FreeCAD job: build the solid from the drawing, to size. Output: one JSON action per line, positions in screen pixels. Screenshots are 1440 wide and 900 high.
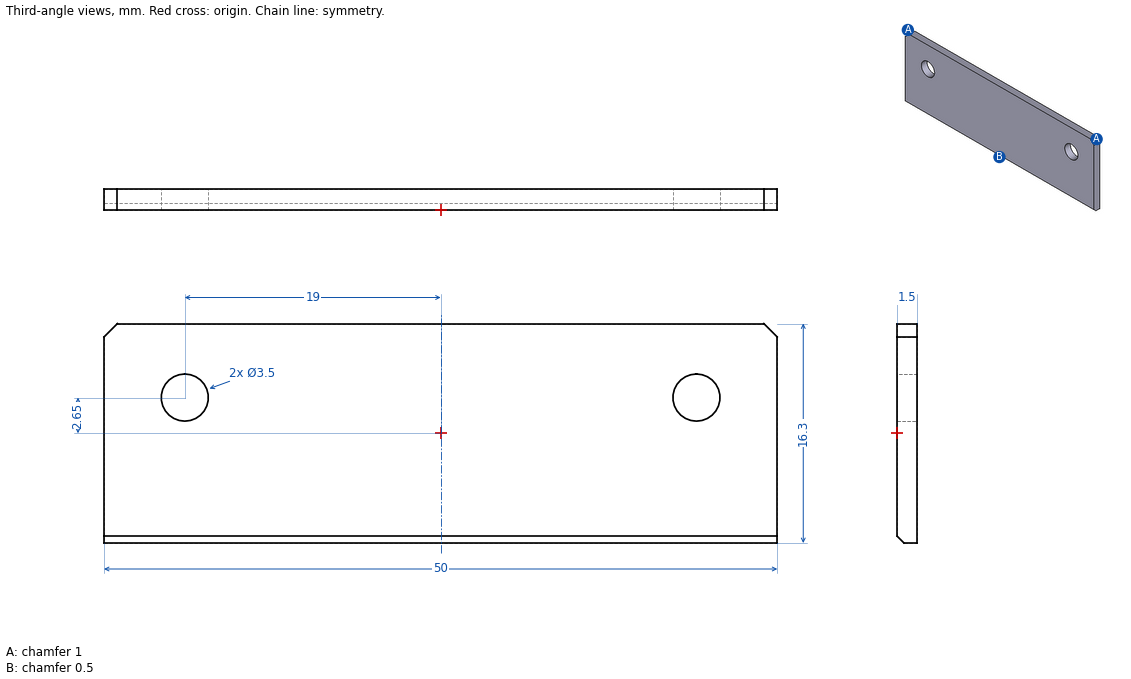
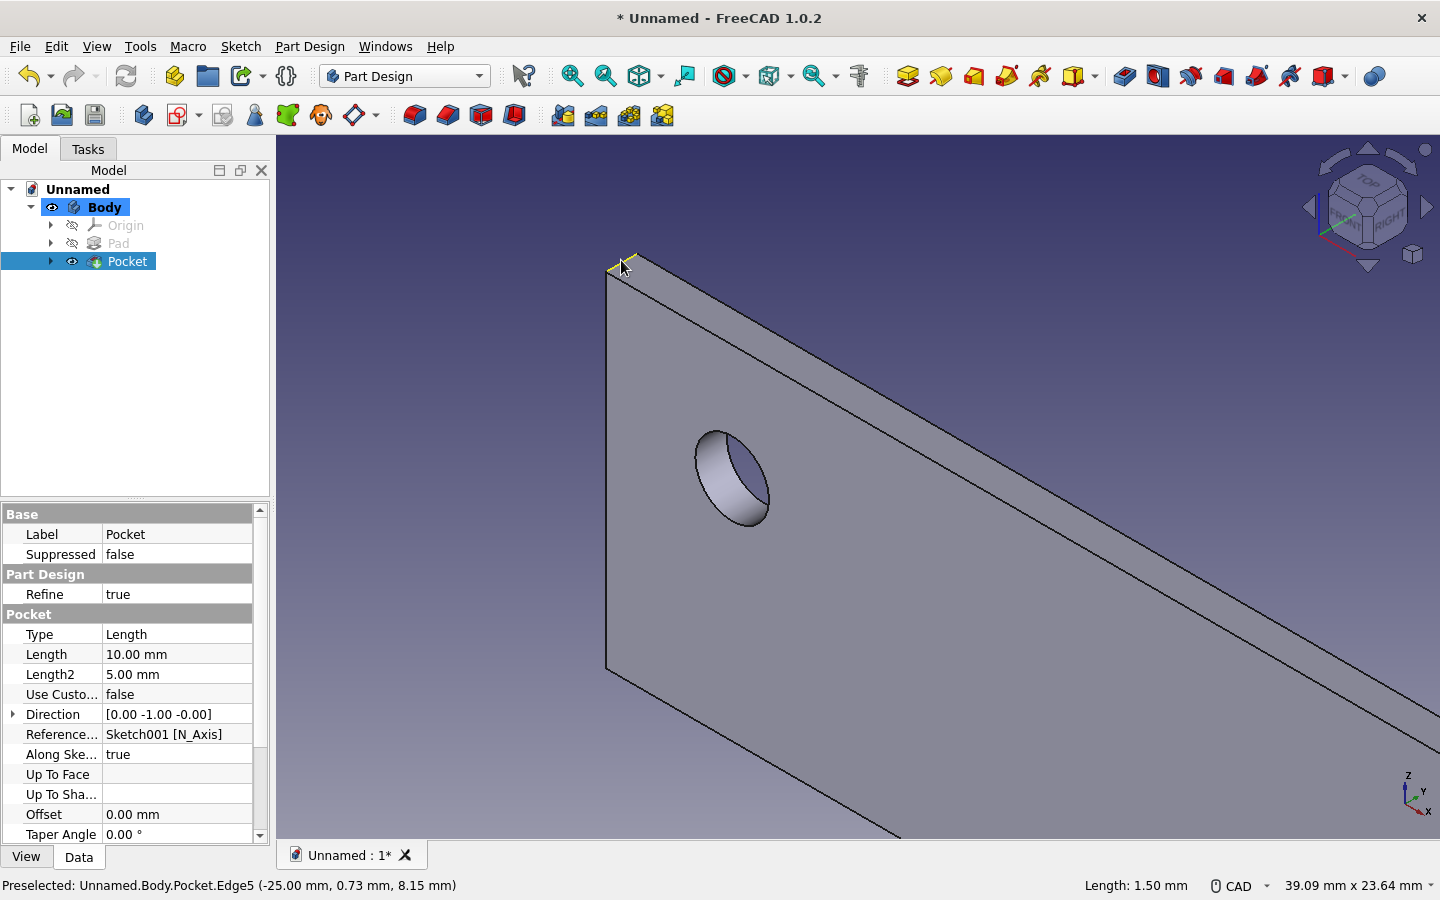
{"action": "key", "text": "v f"}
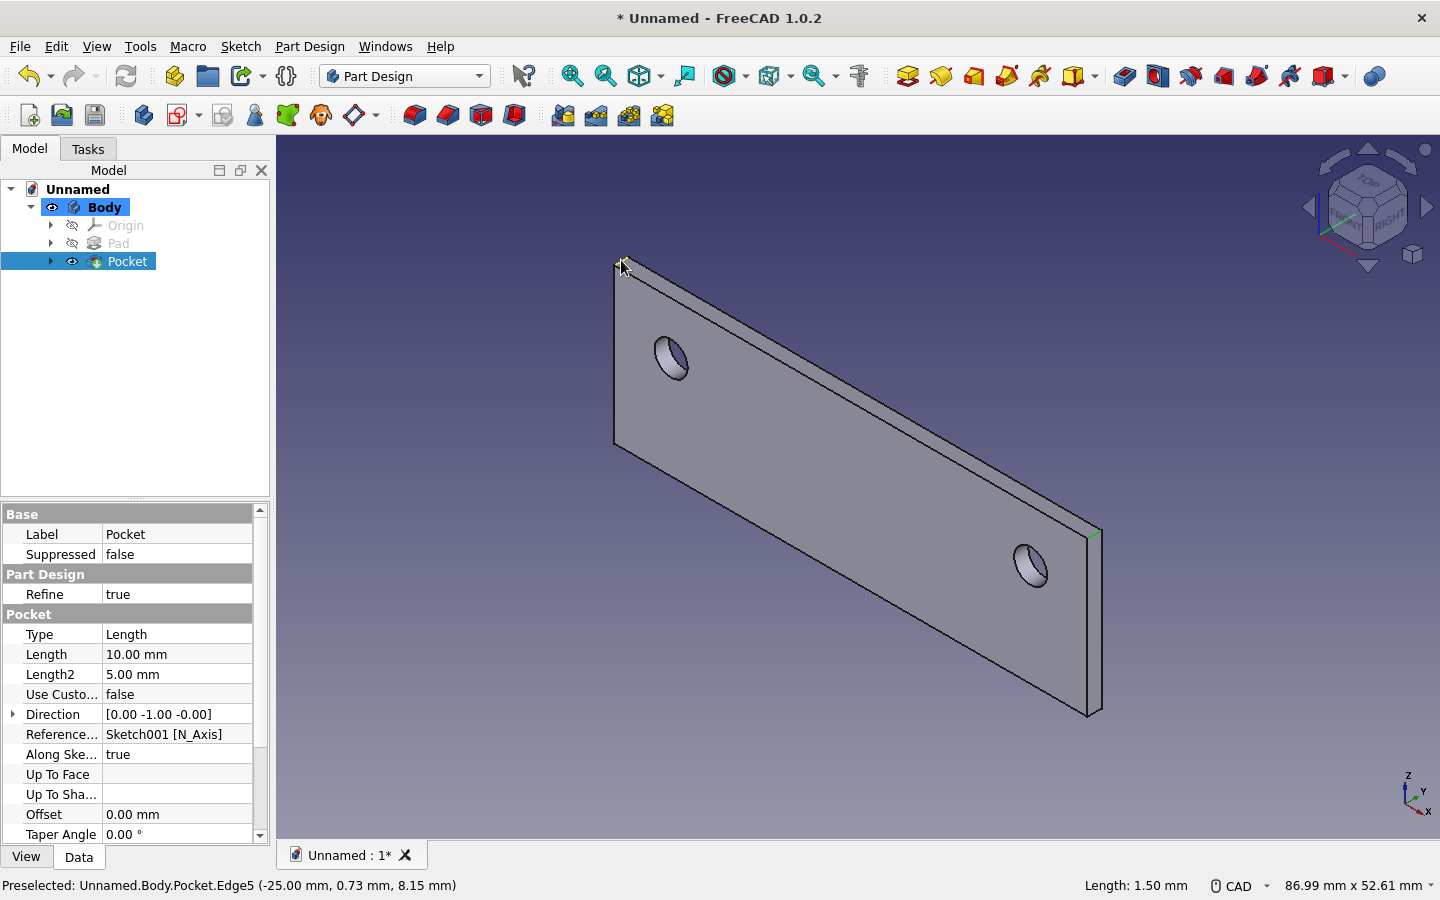
{"action": "key", "text": "2"}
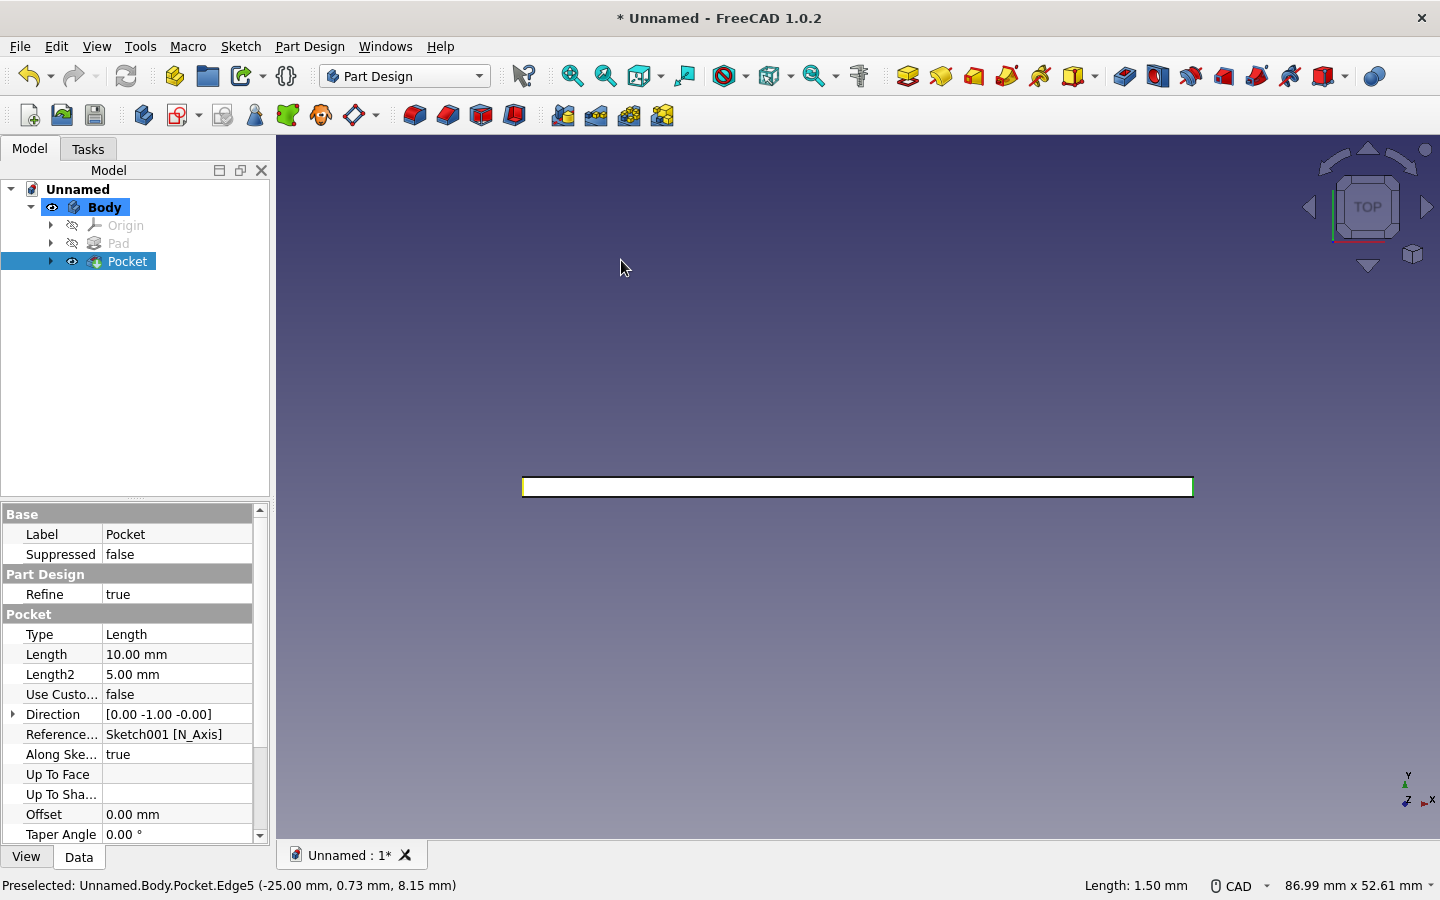
{"action": "left_click", "coordinate": [523, 486], "text": "ctrl"}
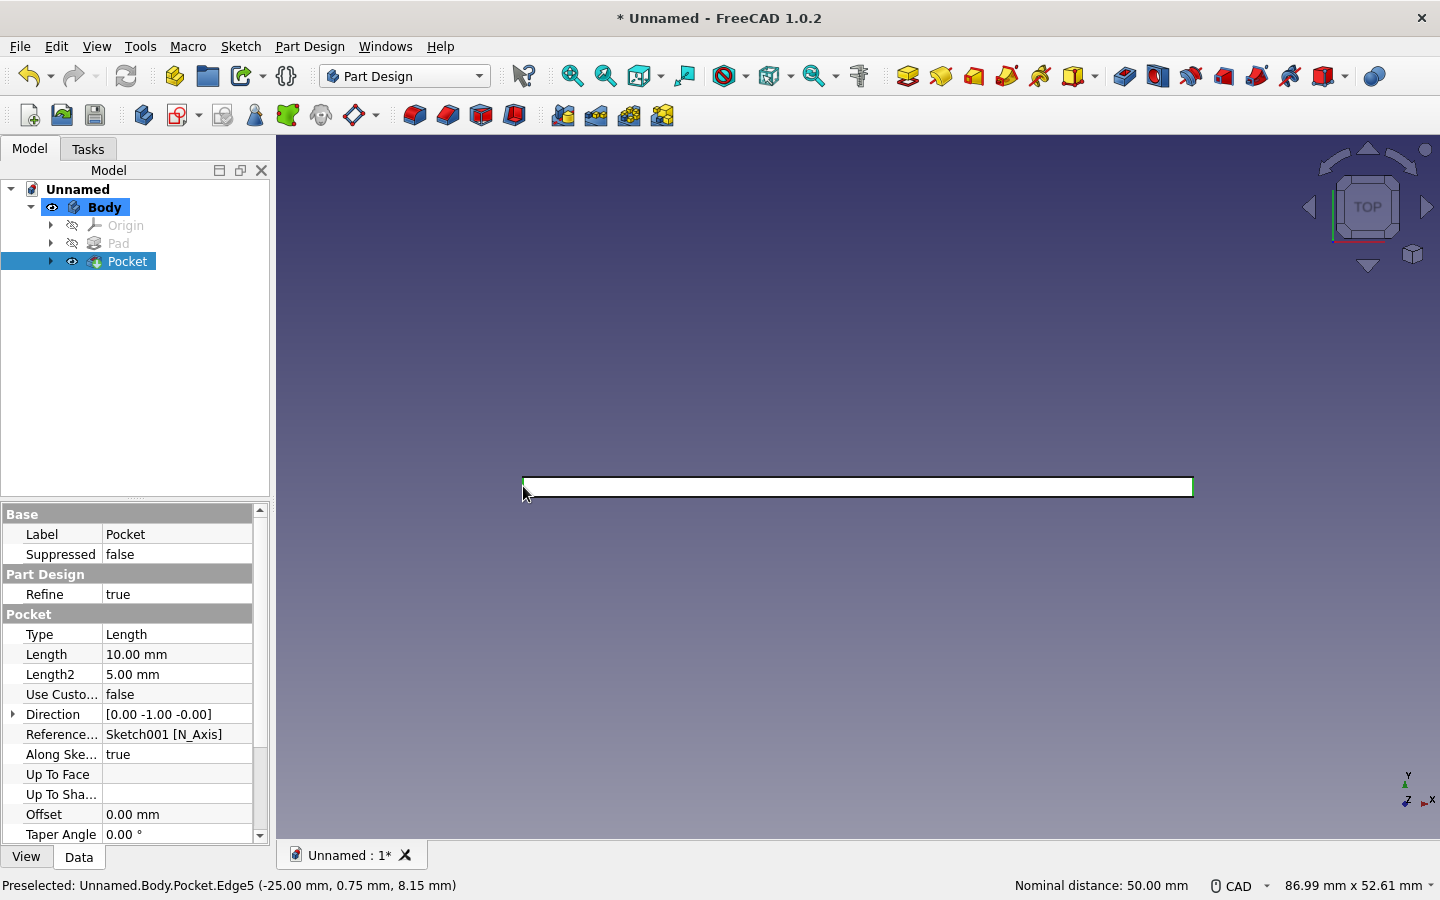
{"action": "left_click", "coordinate": [448, 116]}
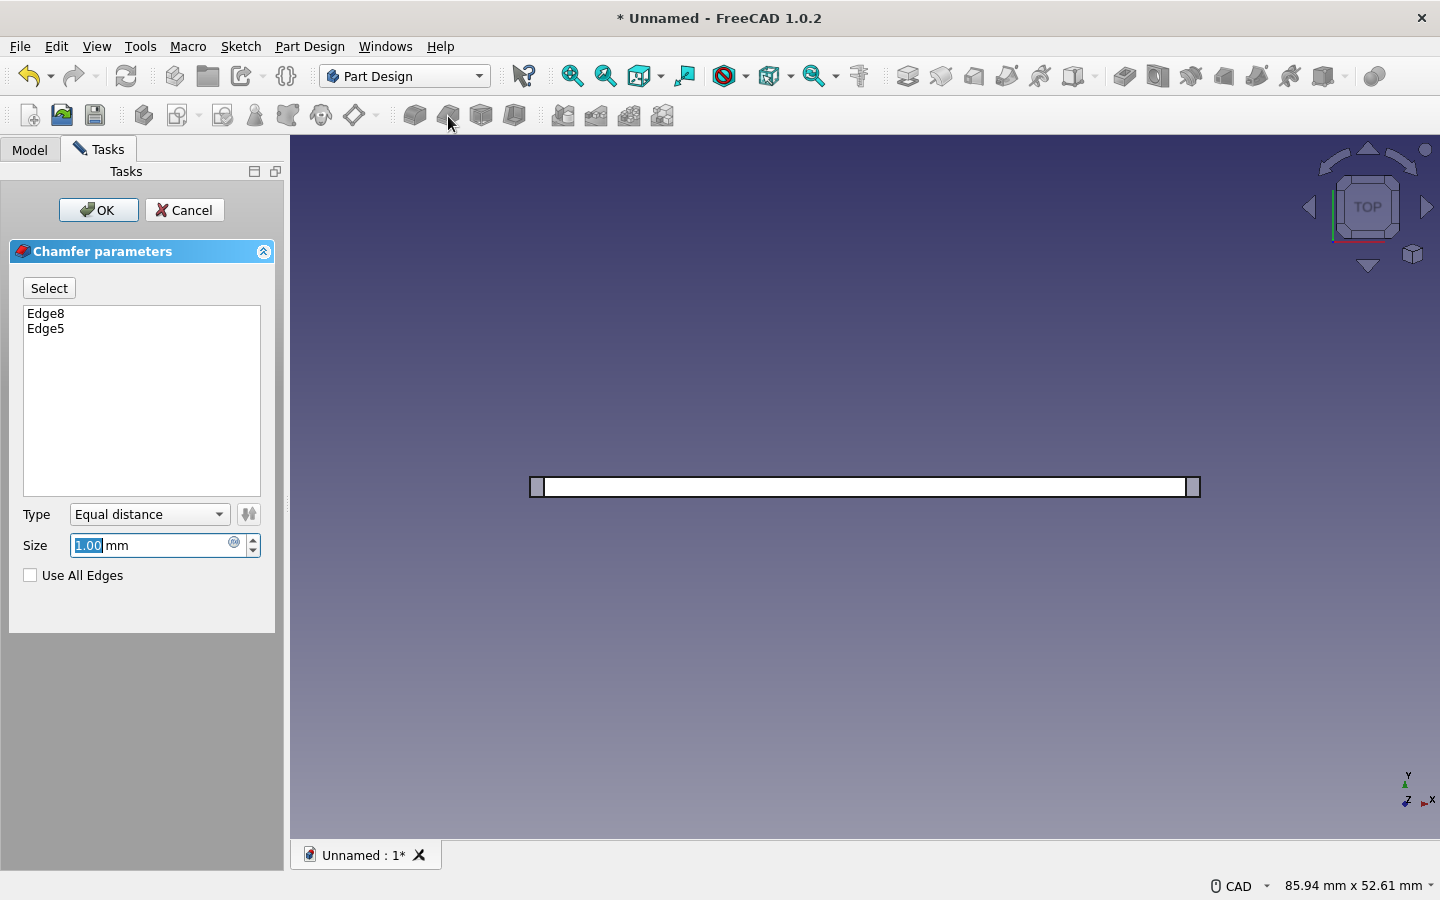
{"action": "type", "text": "1"}
{"action": "key", "text": "Tab"}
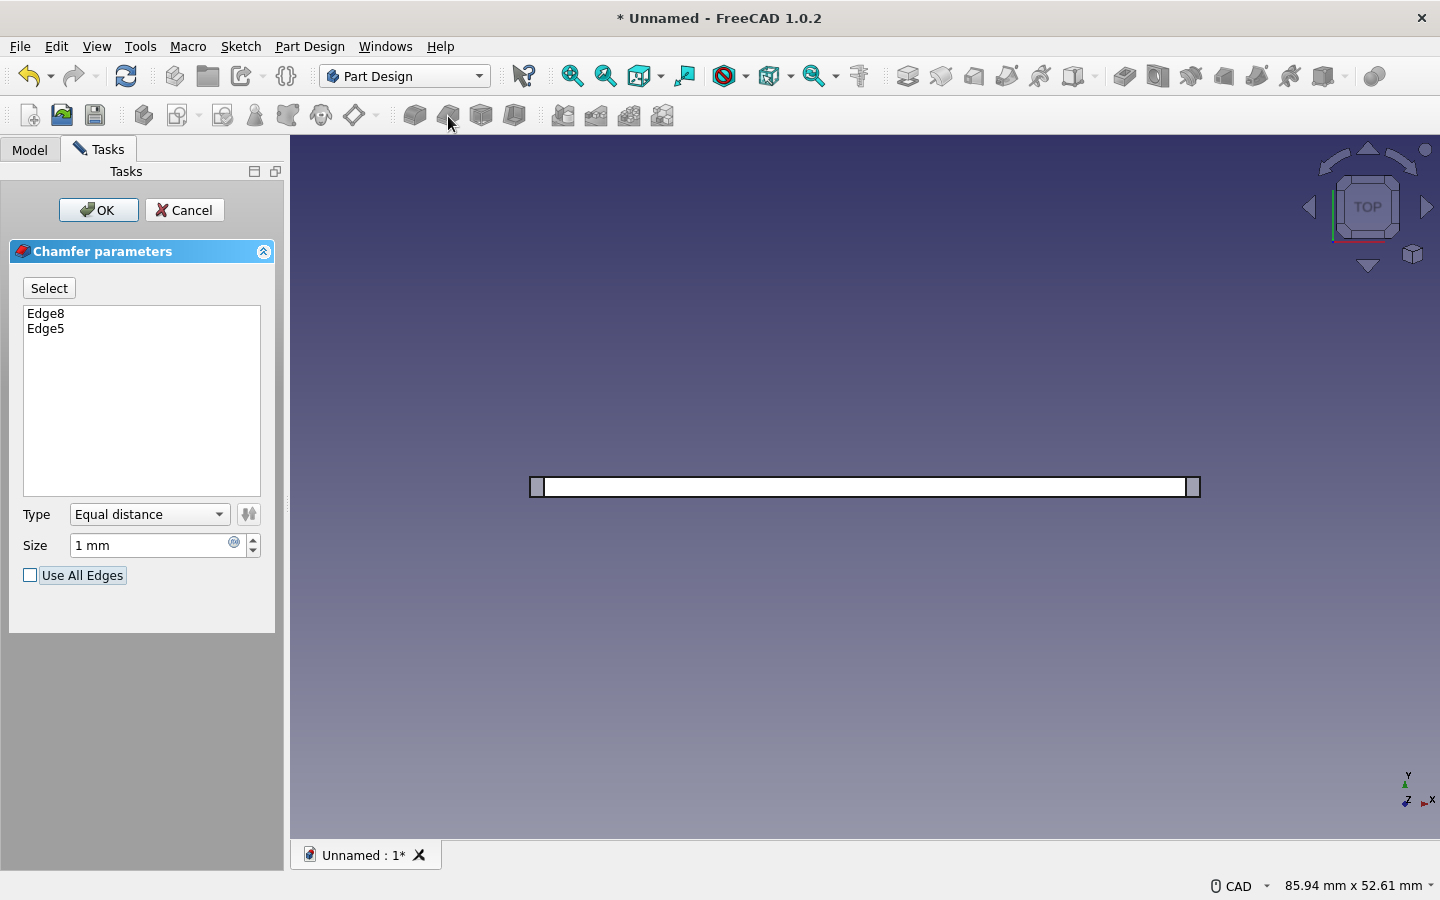
{"action": "left_click", "coordinate": [99, 210]}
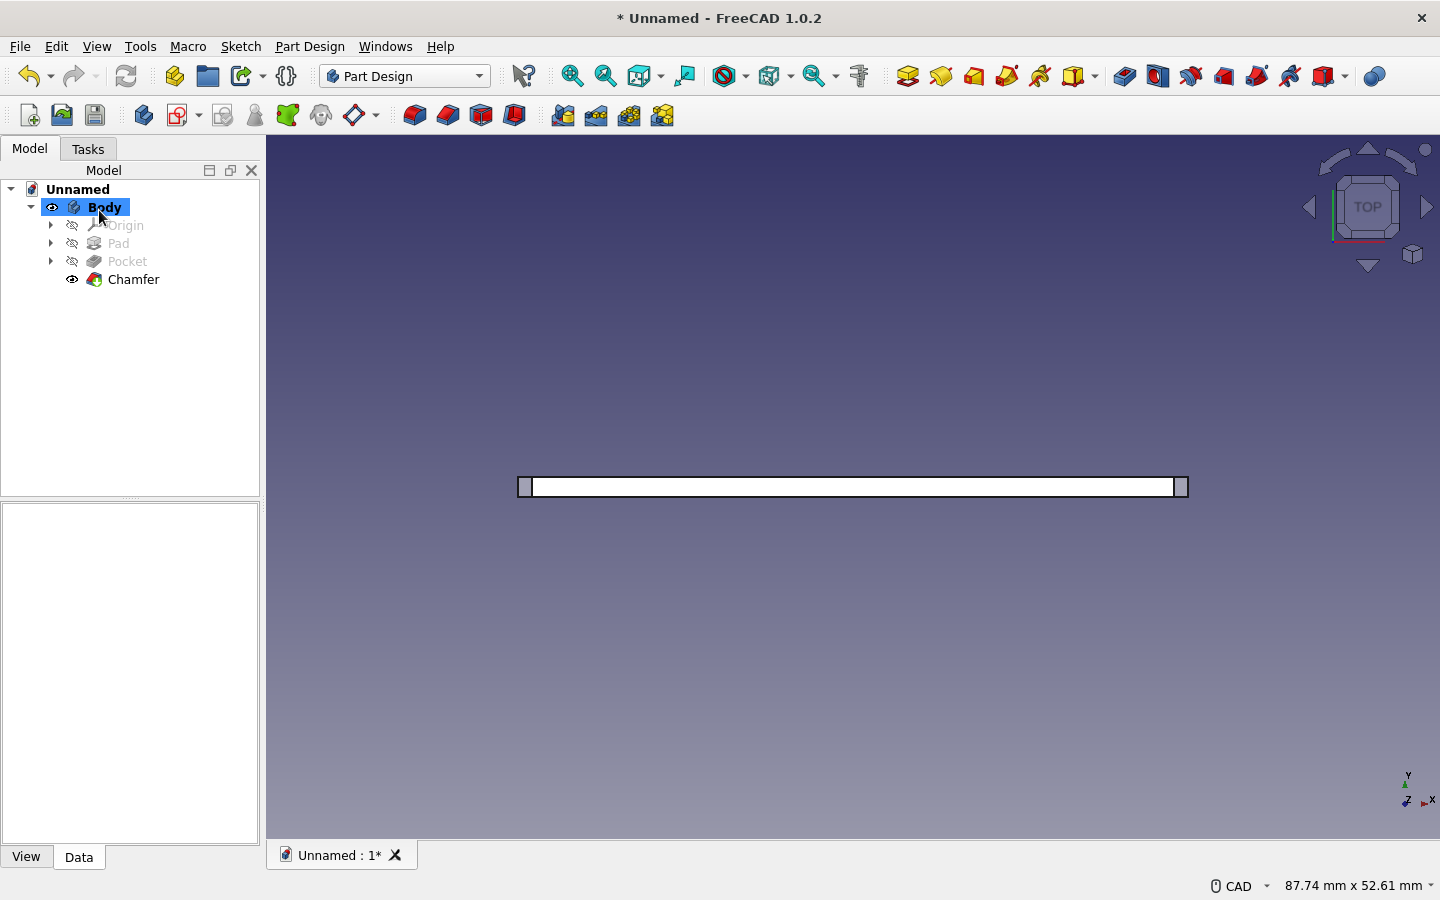
{"action": "key", "text": "0"}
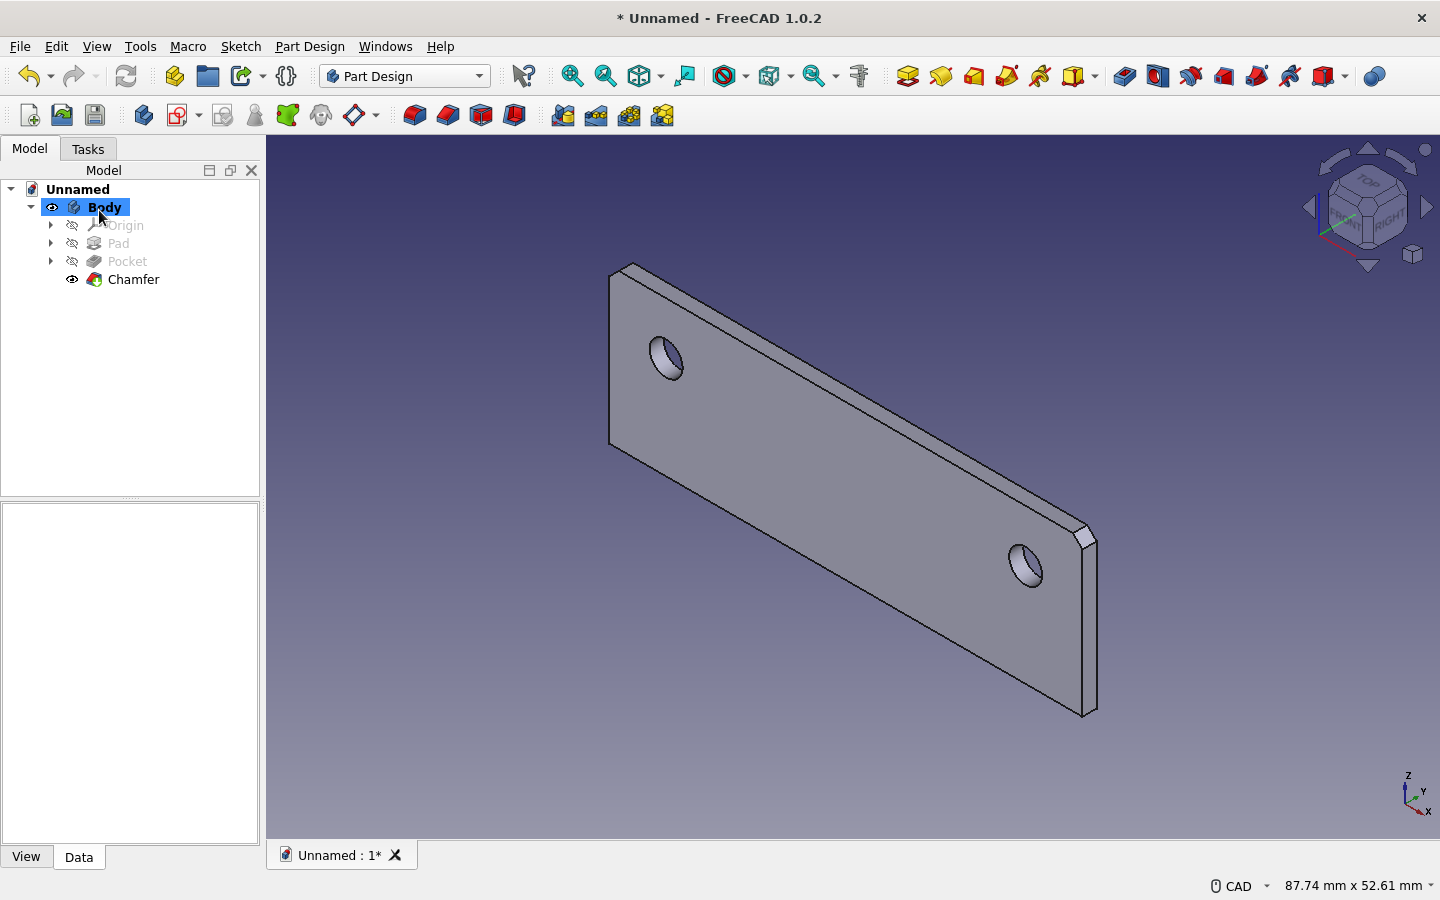
{"action": "key", "text": "2"}